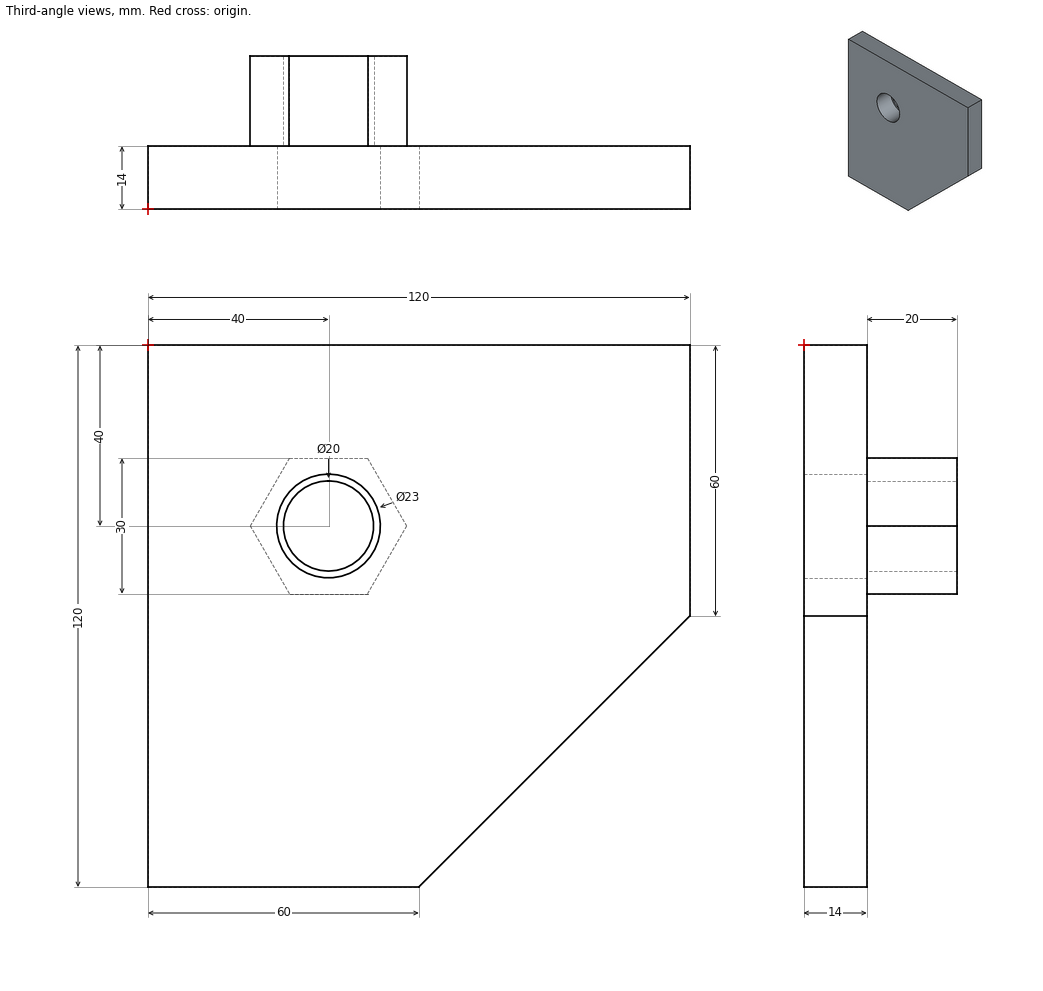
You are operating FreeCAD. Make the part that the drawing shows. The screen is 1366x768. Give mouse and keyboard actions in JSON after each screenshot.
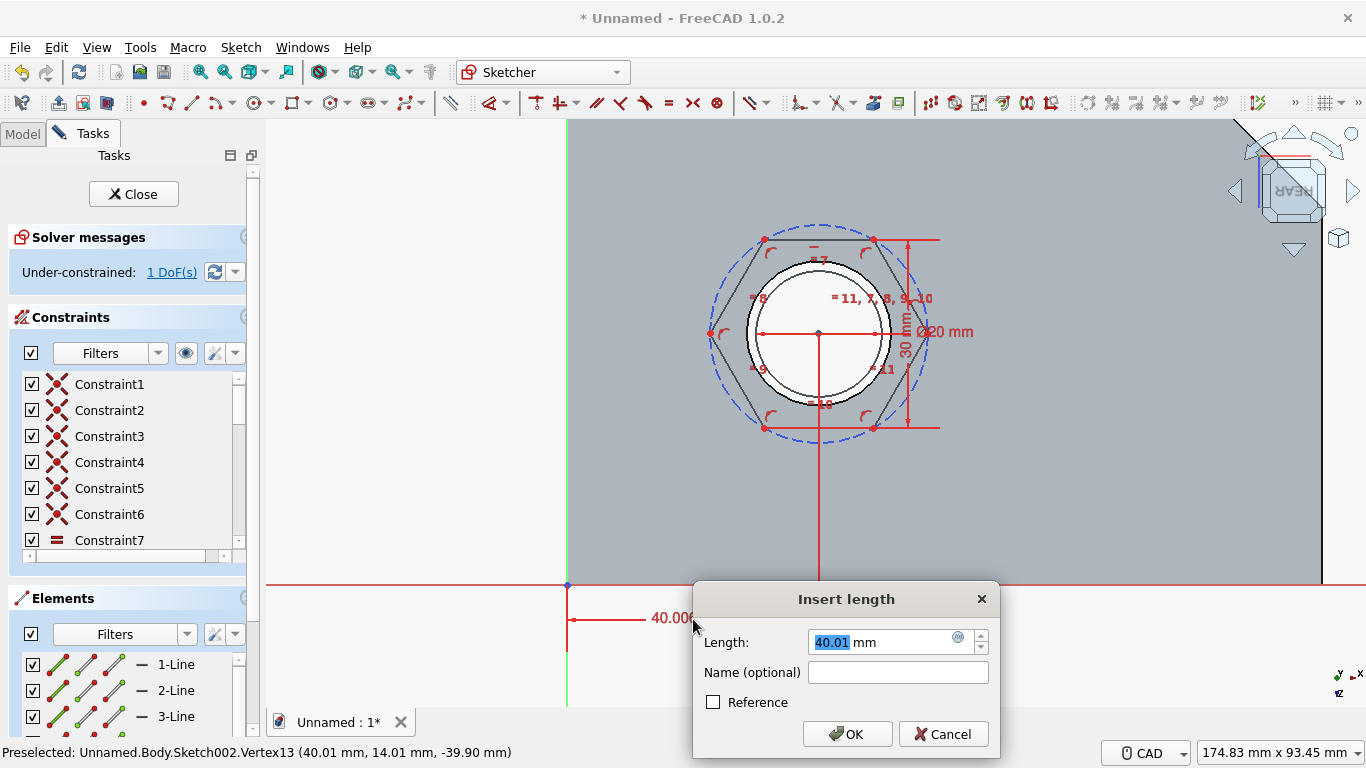
{"action": "type", "text": "40"}
{"action": "key", "text": "Return"}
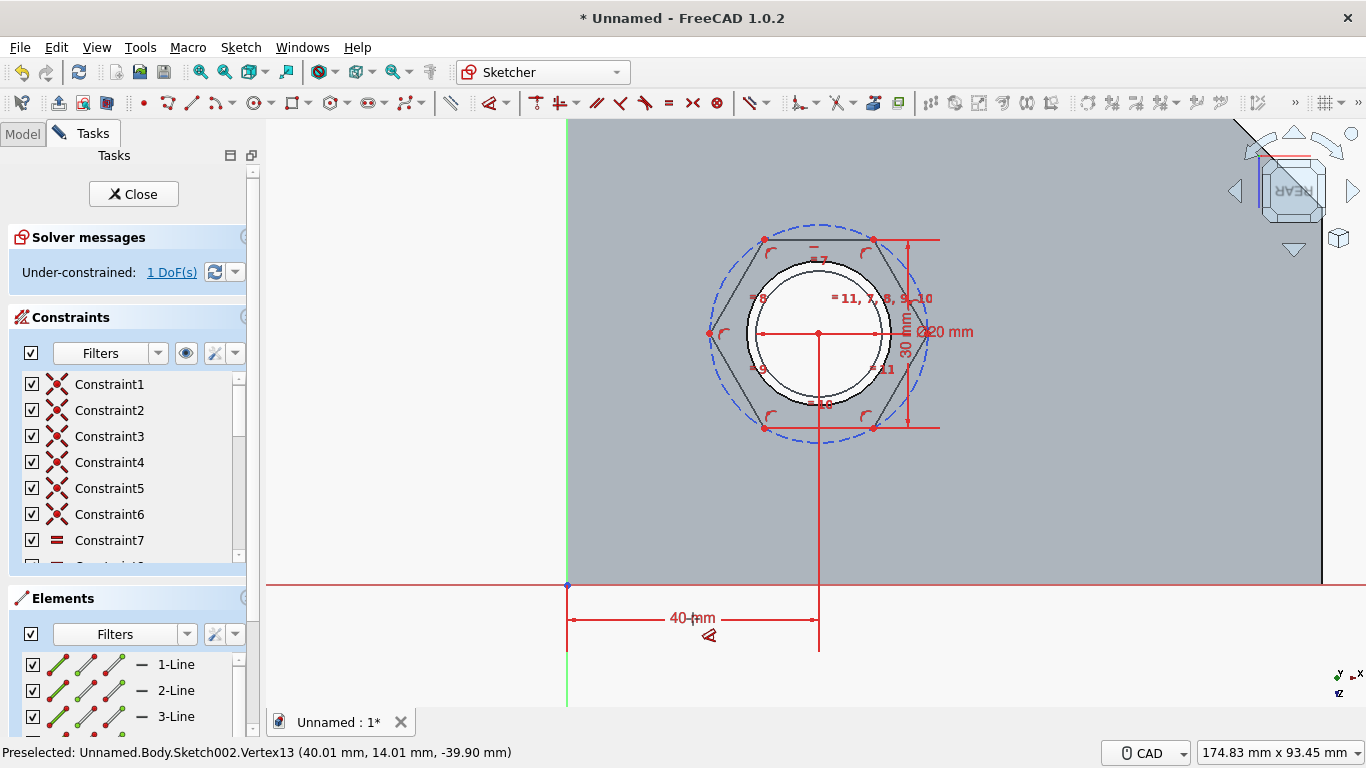
{"action": "left_click", "coordinate": [819, 334]}
{"action": "left_click", "coordinate": [533, 460]}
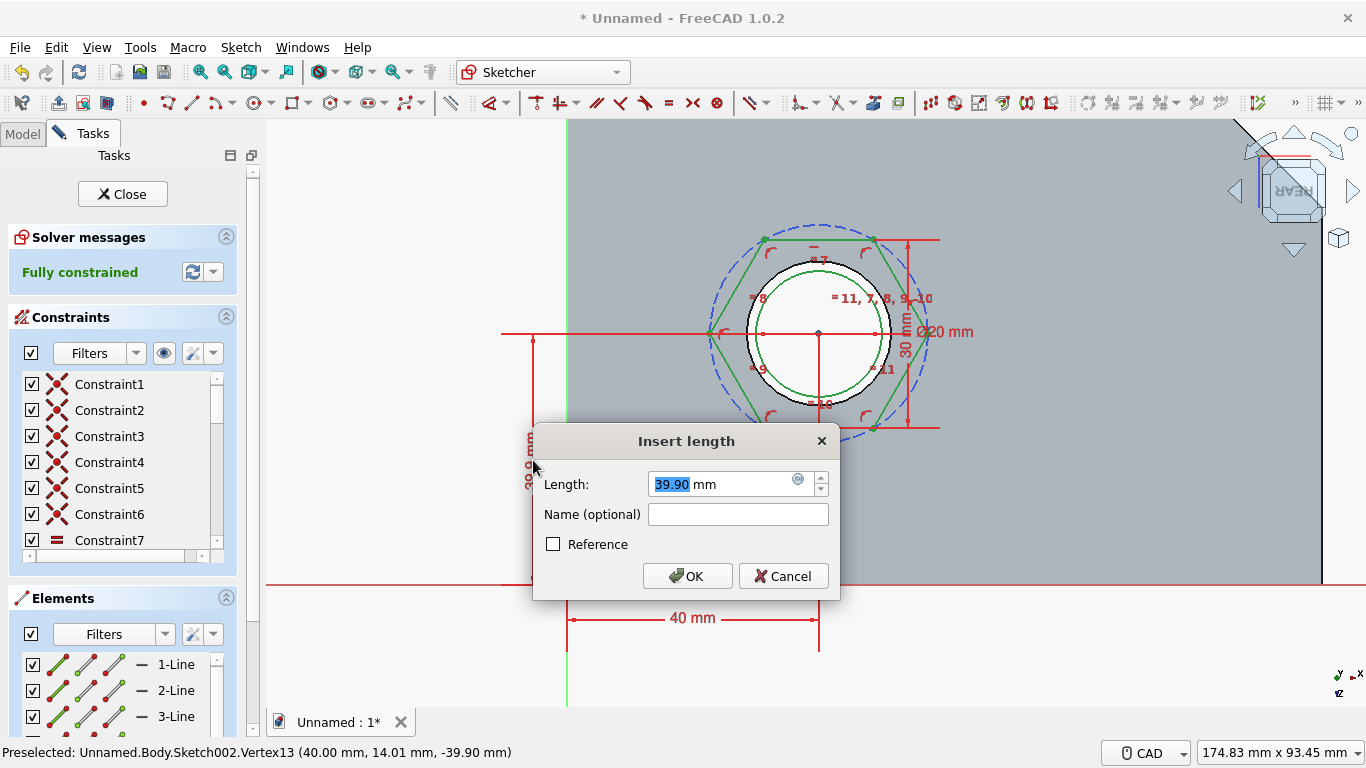
{"action": "type", "text": "40"}
{"action": "key", "text": "Return"}
{"action": "key", "text": "Escape"}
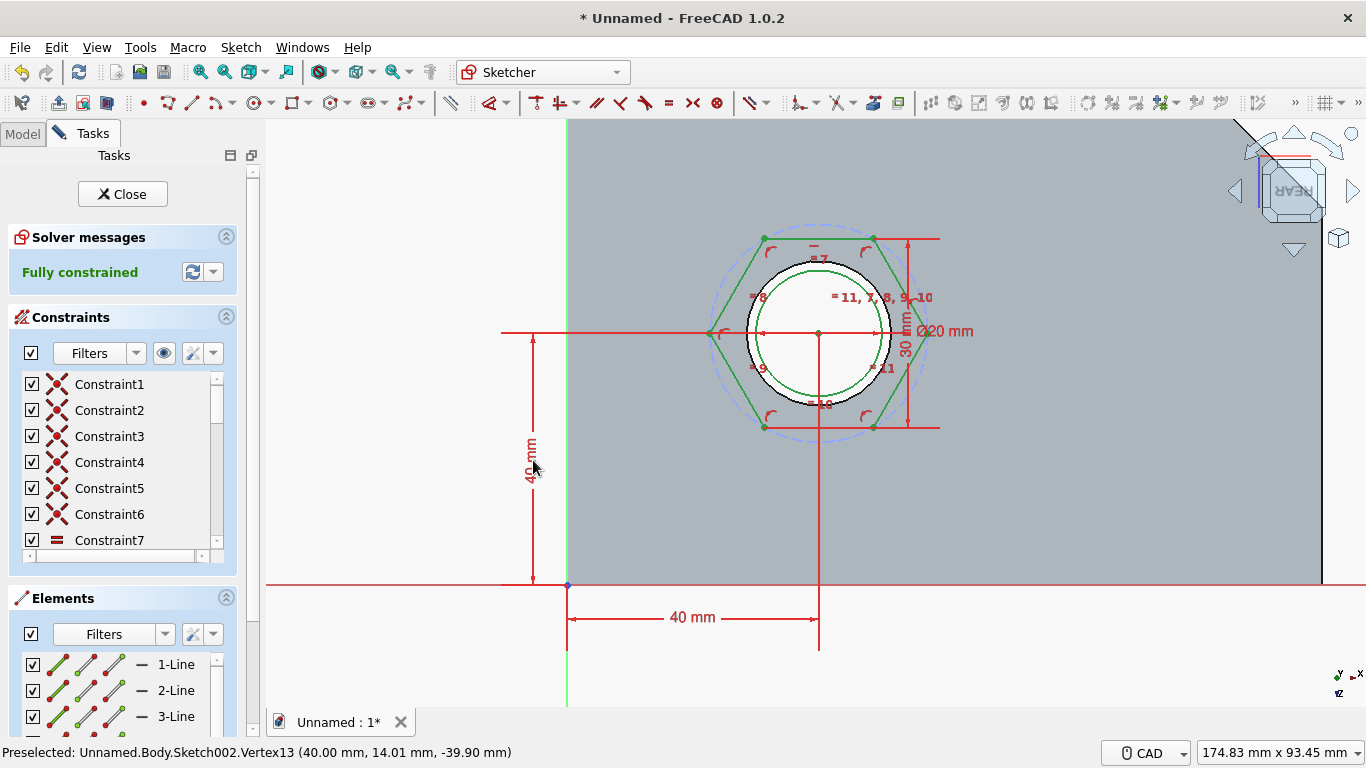
{"action": "left_click", "coordinate": [123, 194]}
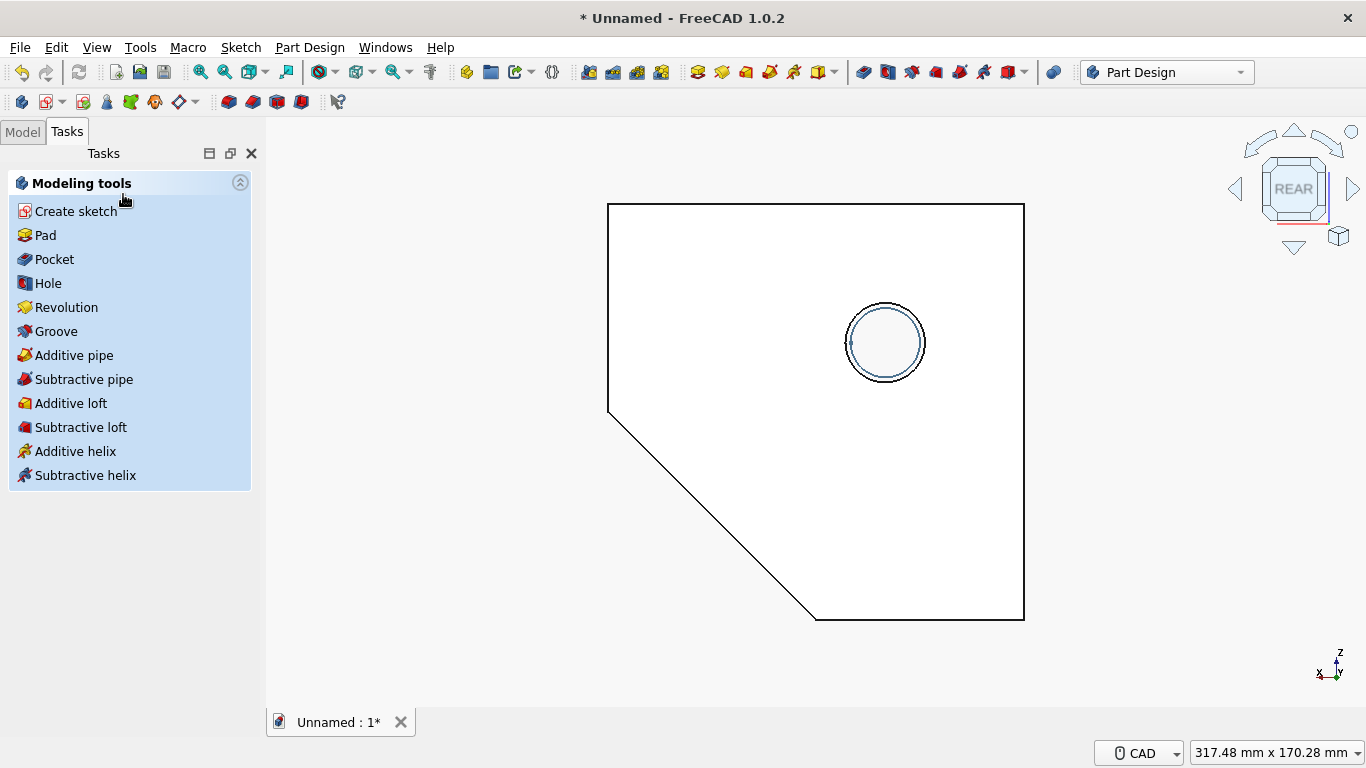
{"action": "left_click", "coordinate": [698, 72]}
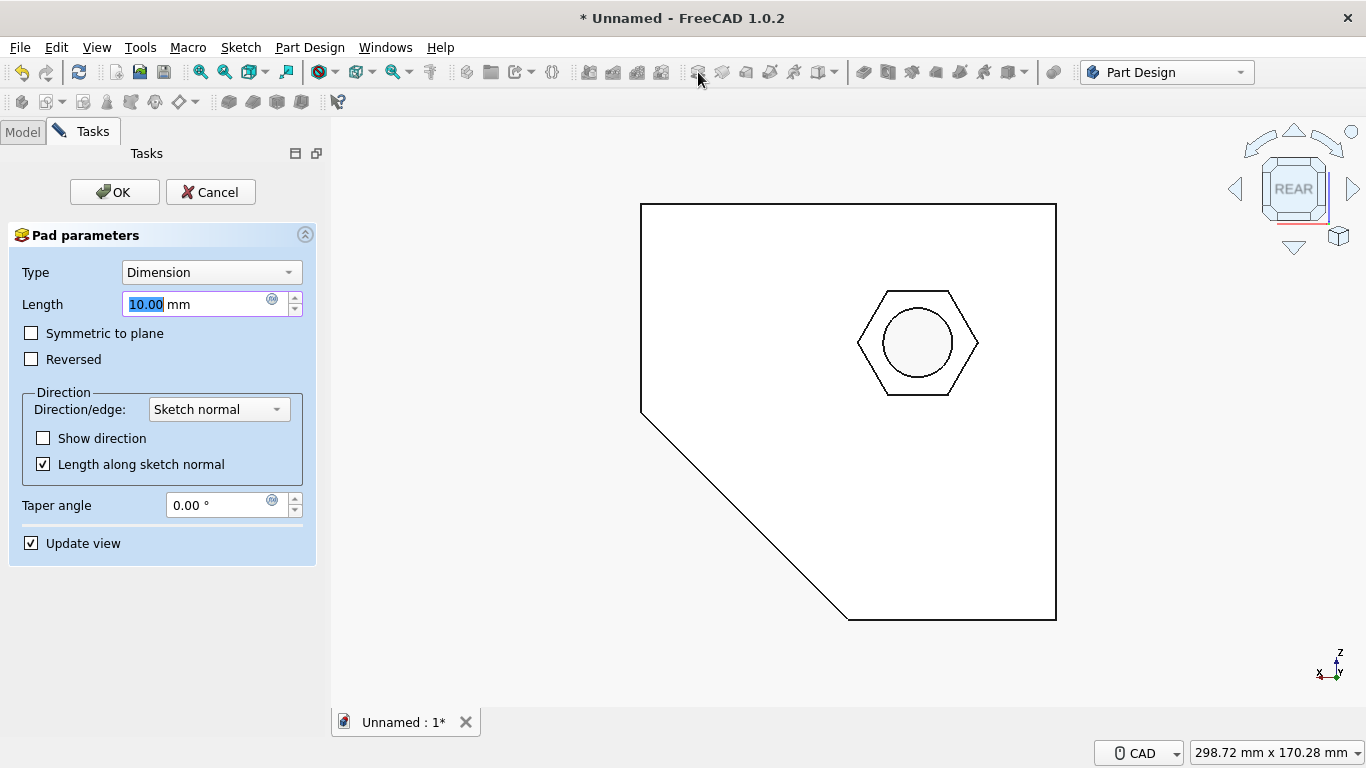
{"action": "type", "text": "20"}
{"action": "key", "text": "Tab"}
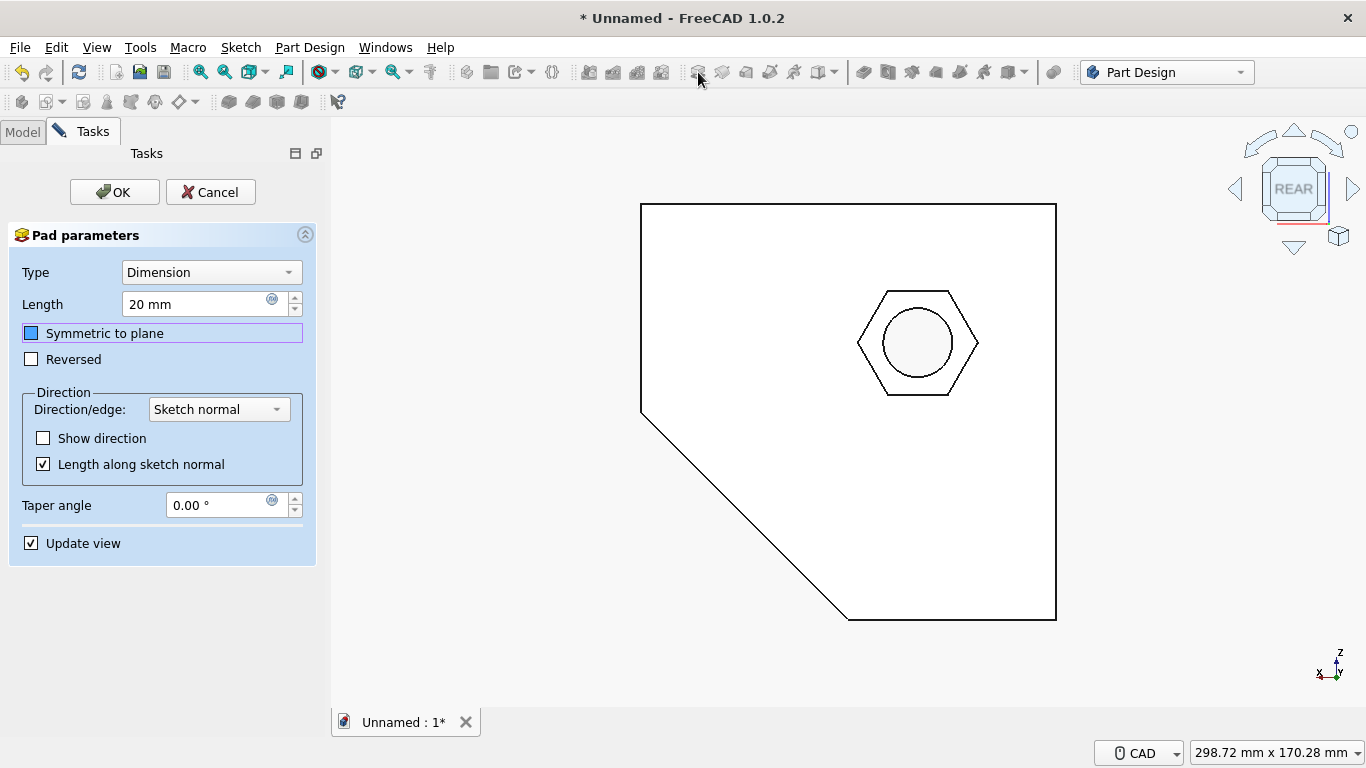
{"action": "left_click", "coordinate": [115, 192]}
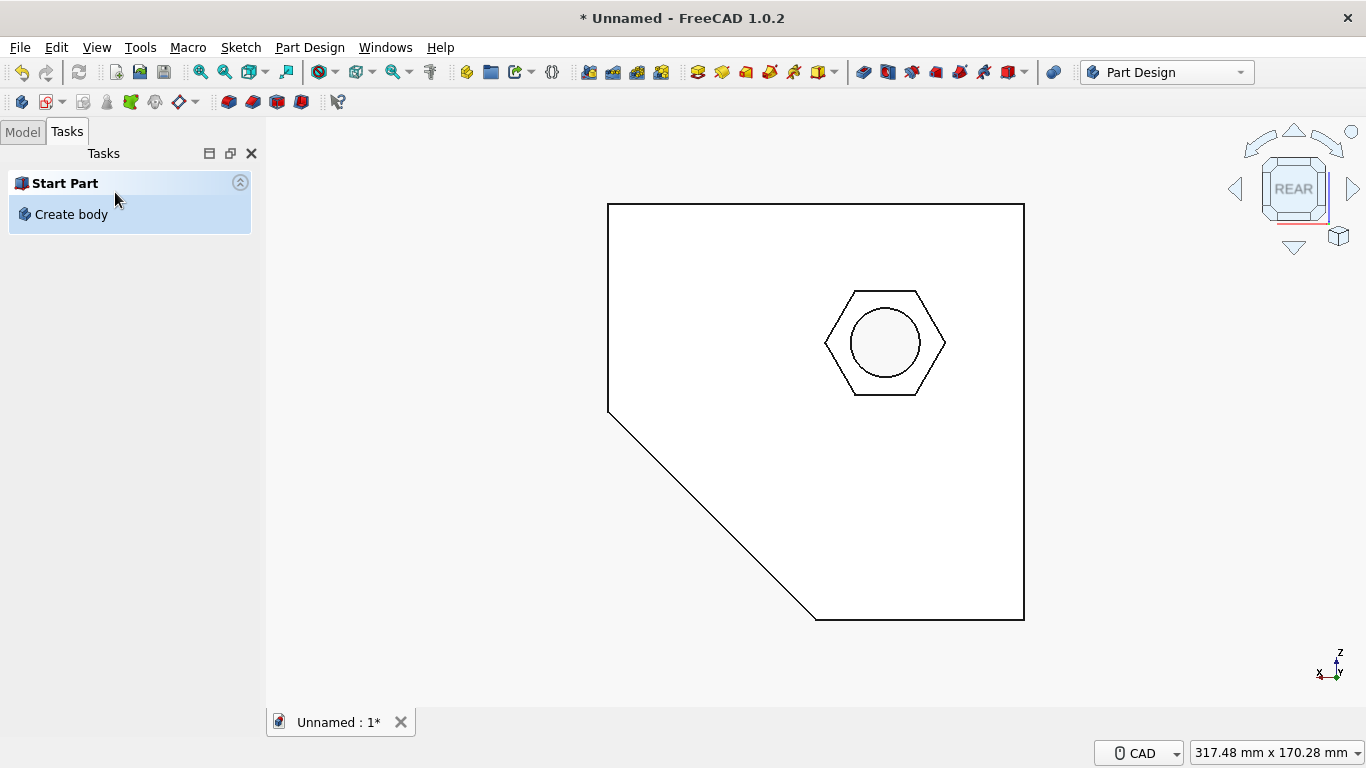
{"action": "key", "text": "0"}